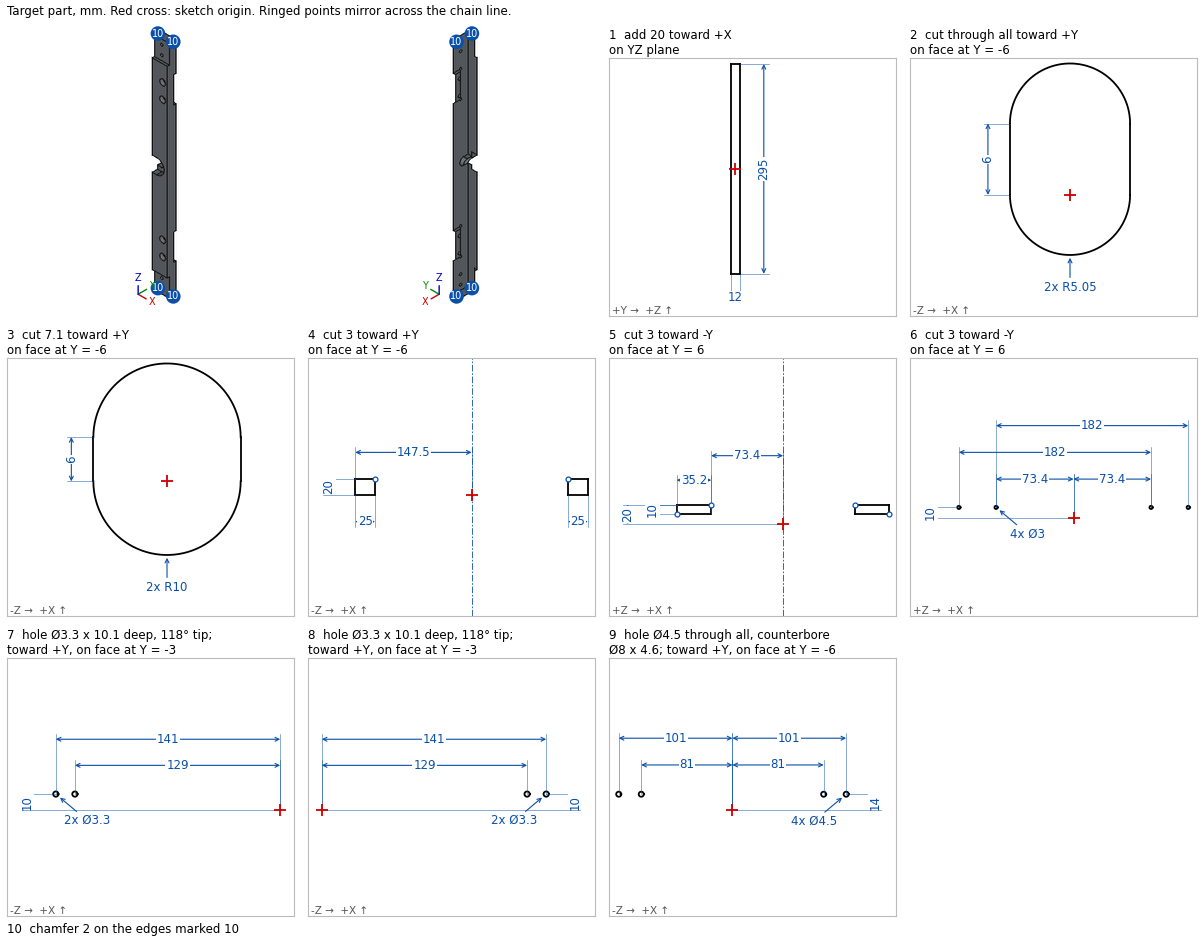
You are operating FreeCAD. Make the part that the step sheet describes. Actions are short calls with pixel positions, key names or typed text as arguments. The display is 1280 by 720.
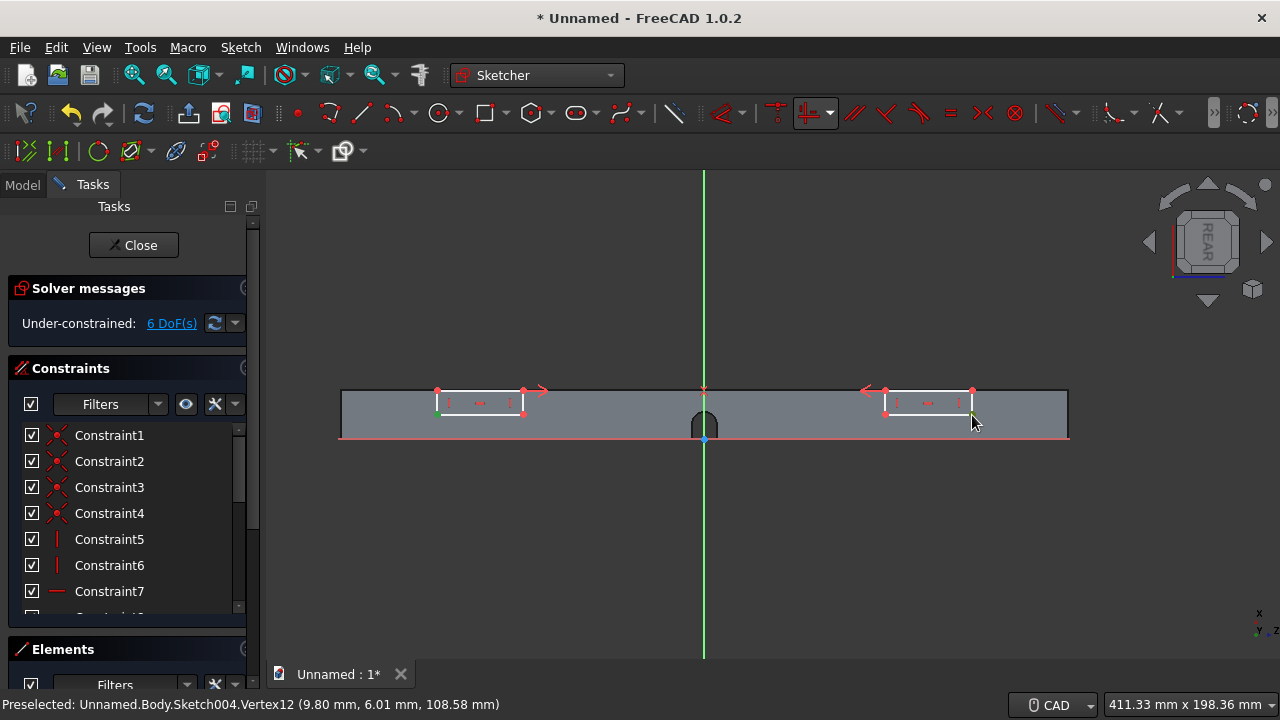
click(704, 600)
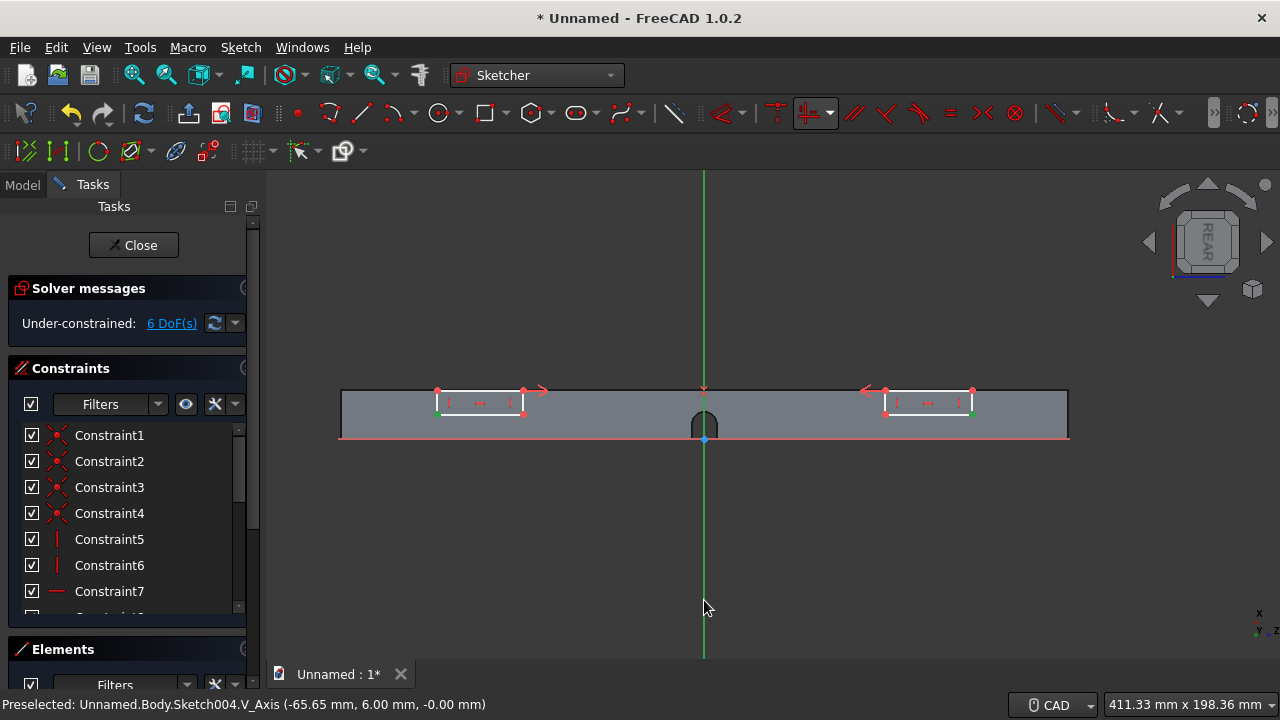
click(984, 114)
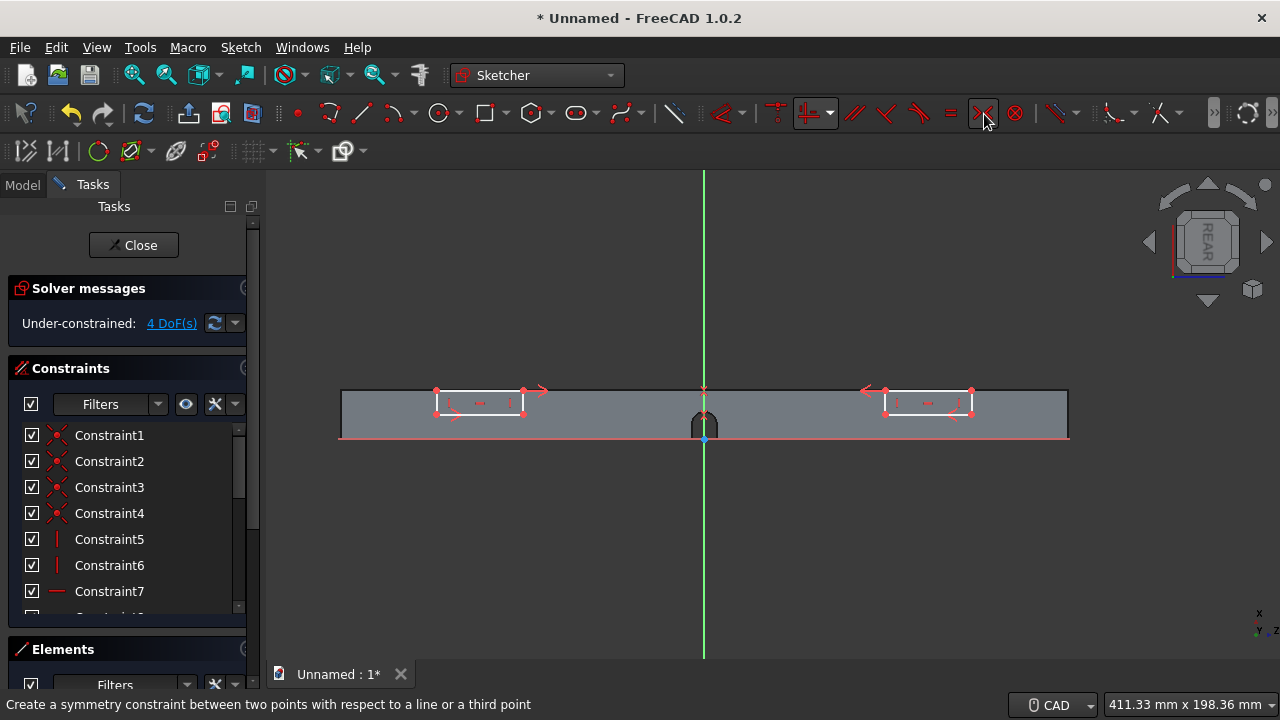
click(722, 114)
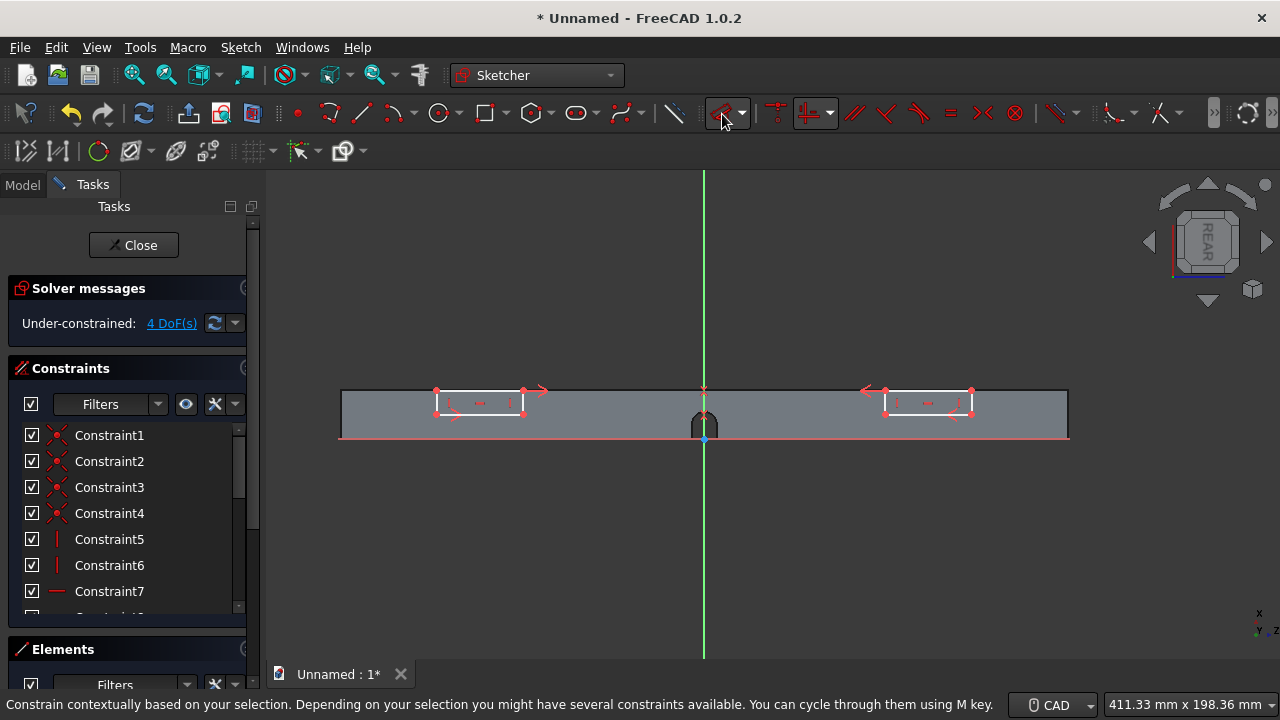
scroll(437, 401, up, 3)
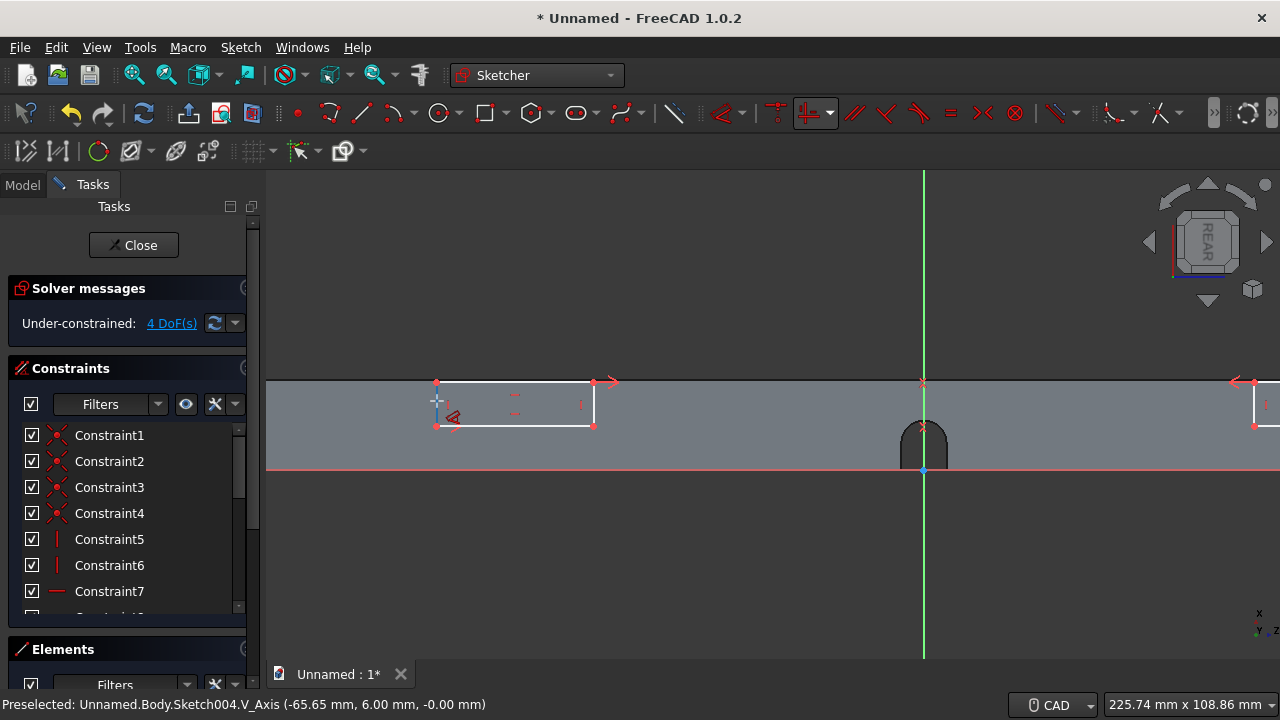
click(437, 400)
click(403, 404)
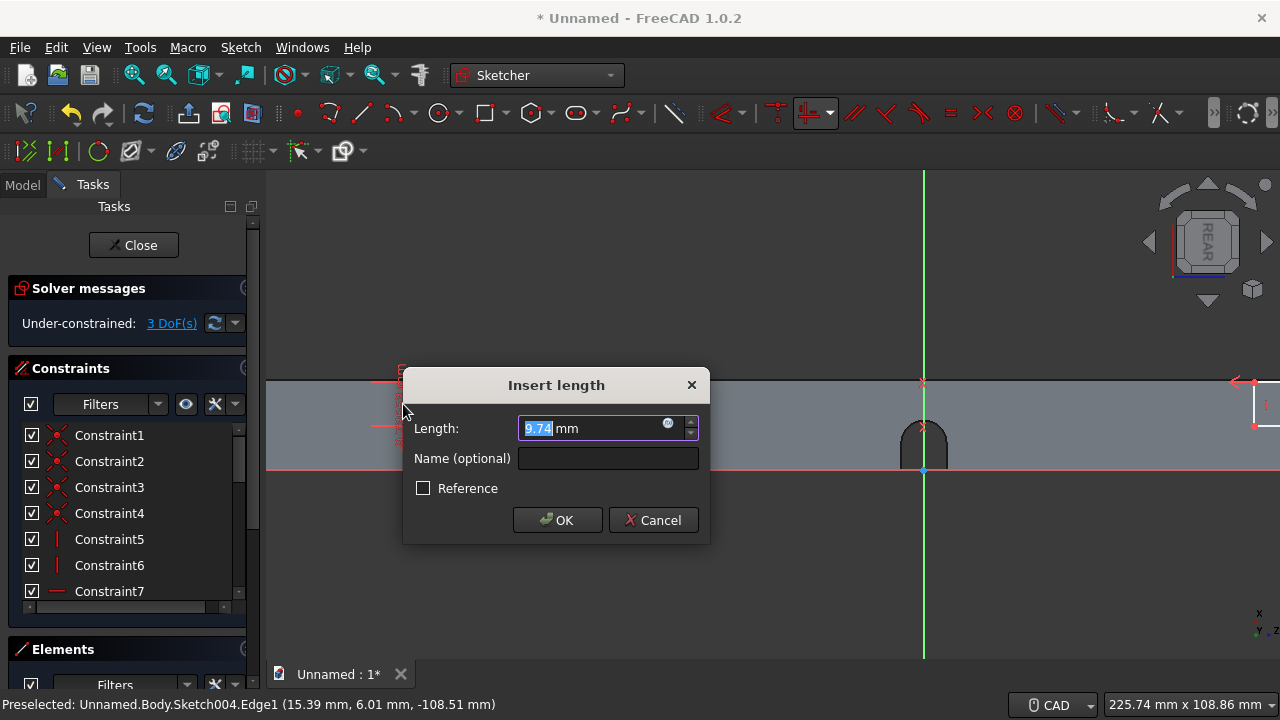
text(10)
key(Return)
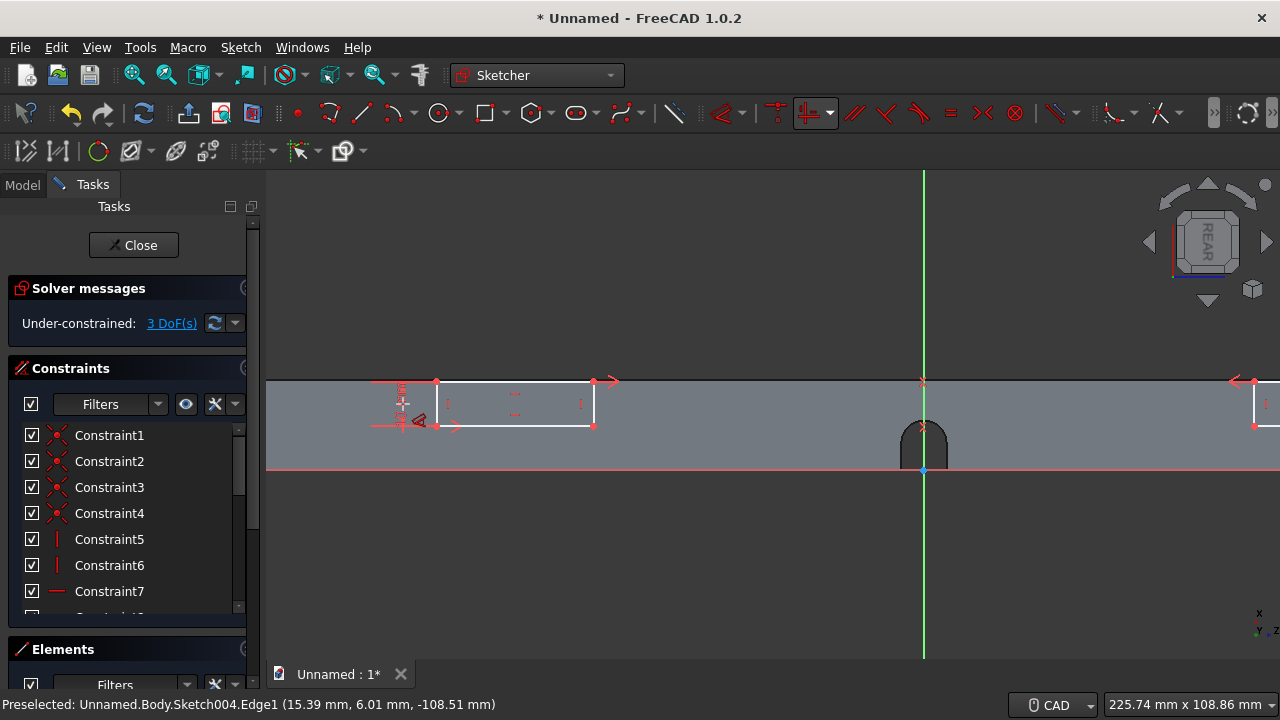
click(437, 382)
click(403, 426)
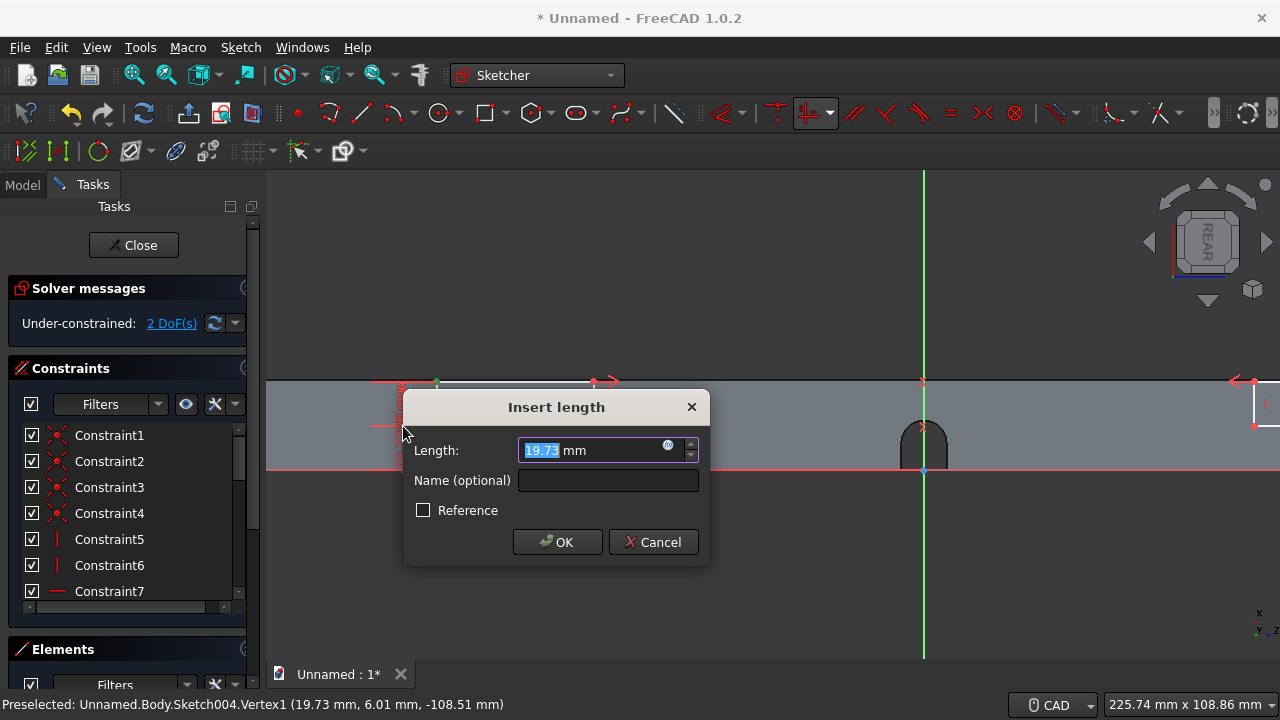
text(20)
key(Return)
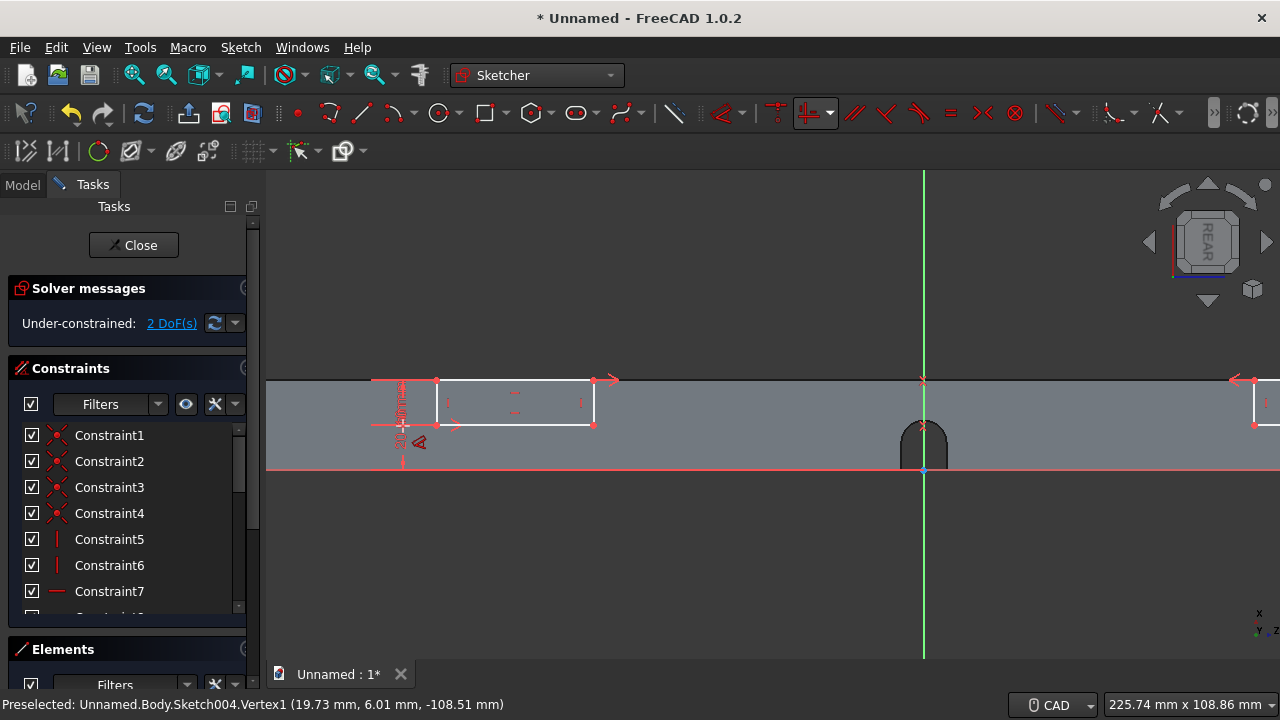
click(484, 425)
click(515, 367)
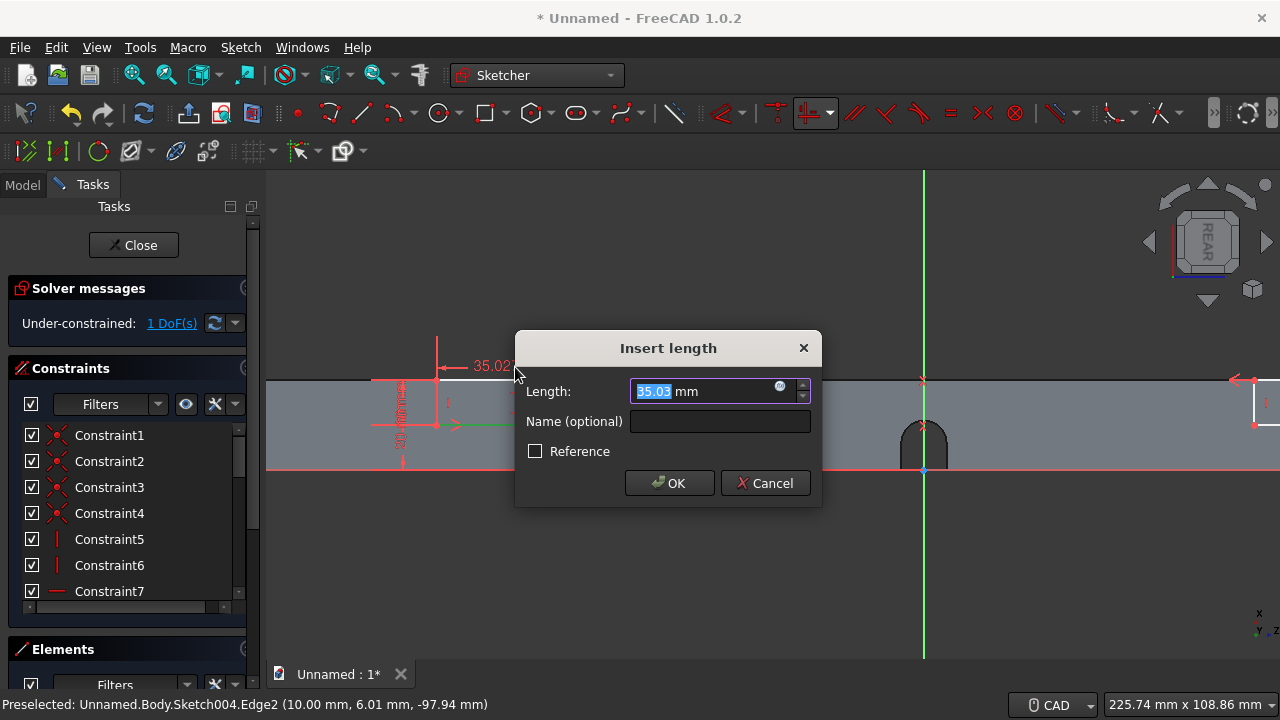
text(35.2)
key(Return)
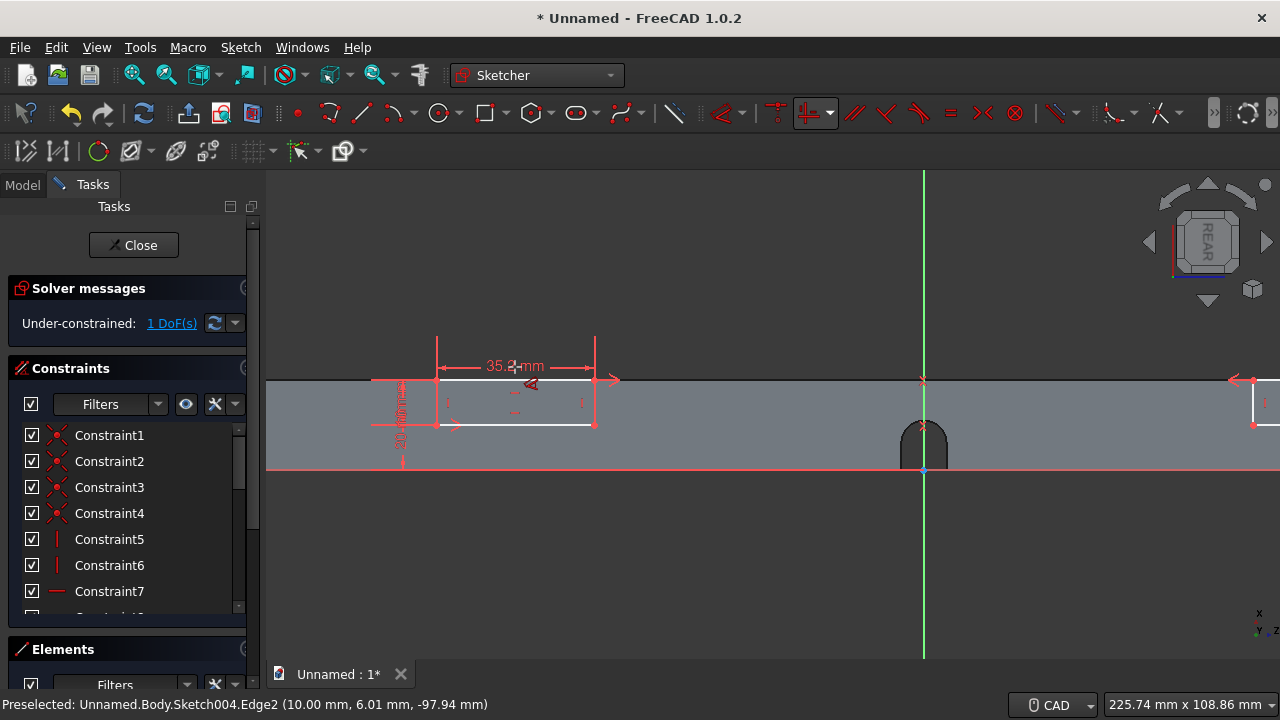
click(595, 425)
click(759, 504)